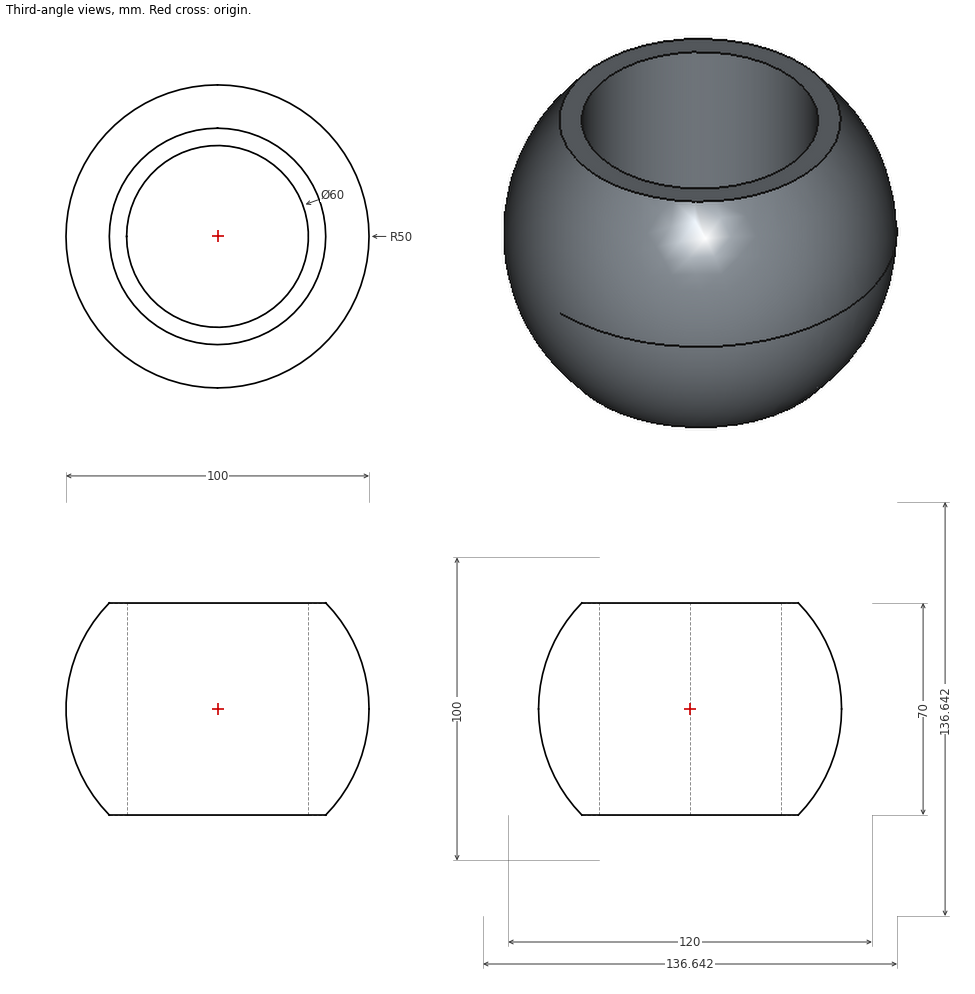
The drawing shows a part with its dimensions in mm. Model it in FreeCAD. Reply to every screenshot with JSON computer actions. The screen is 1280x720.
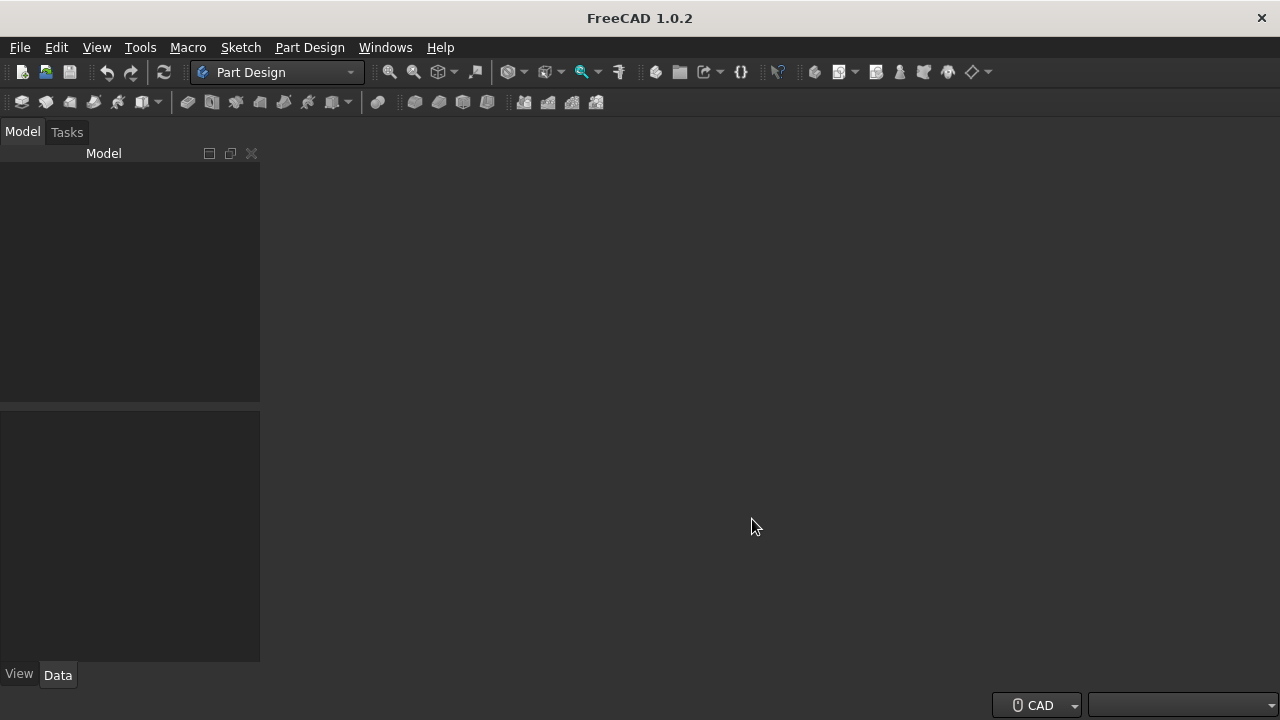
{"action": "left_click", "coordinate": [22, 72]}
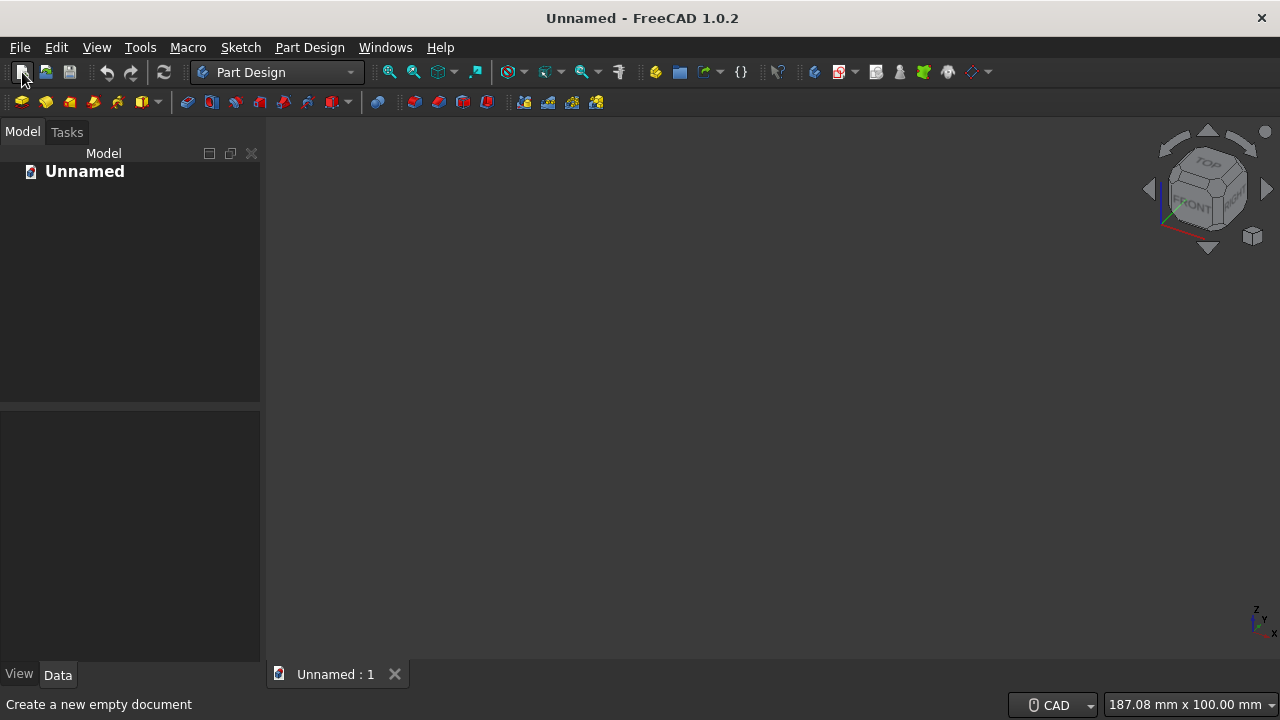
{"action": "left_click", "coordinate": [840, 72]}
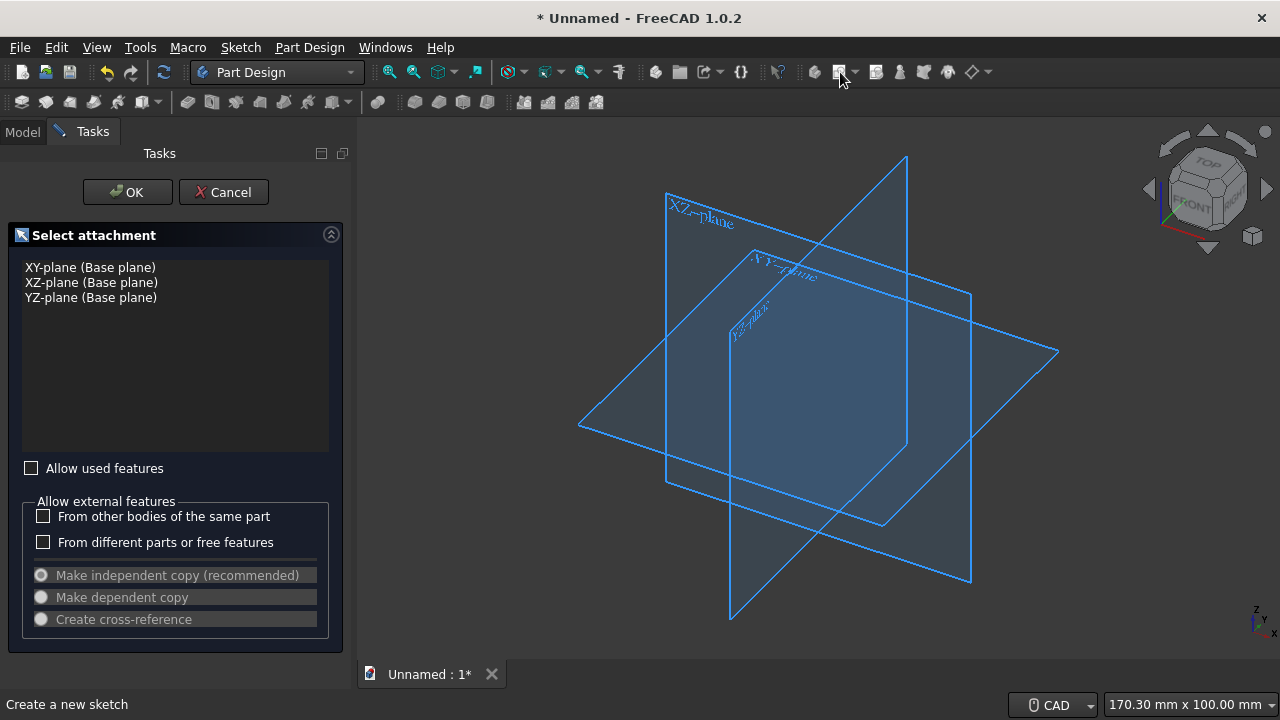
{"action": "left_click", "coordinate": [82, 268]}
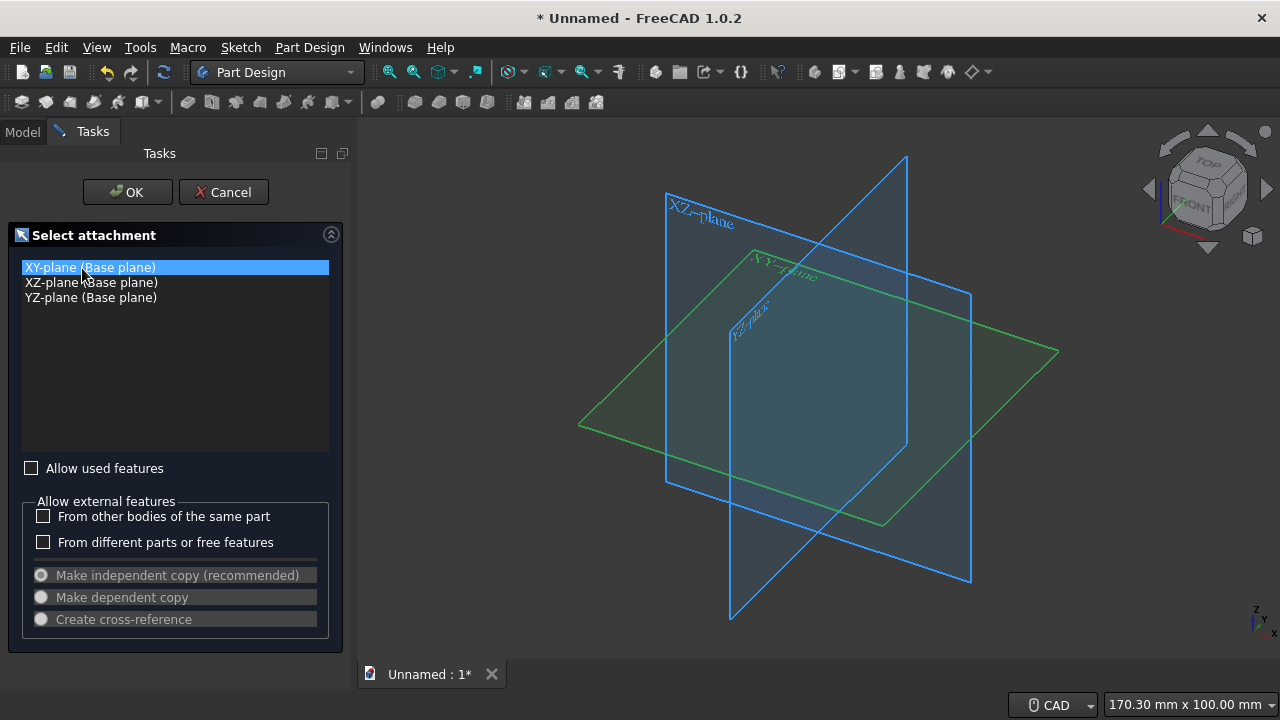
{"action": "left_click", "coordinate": [128, 192]}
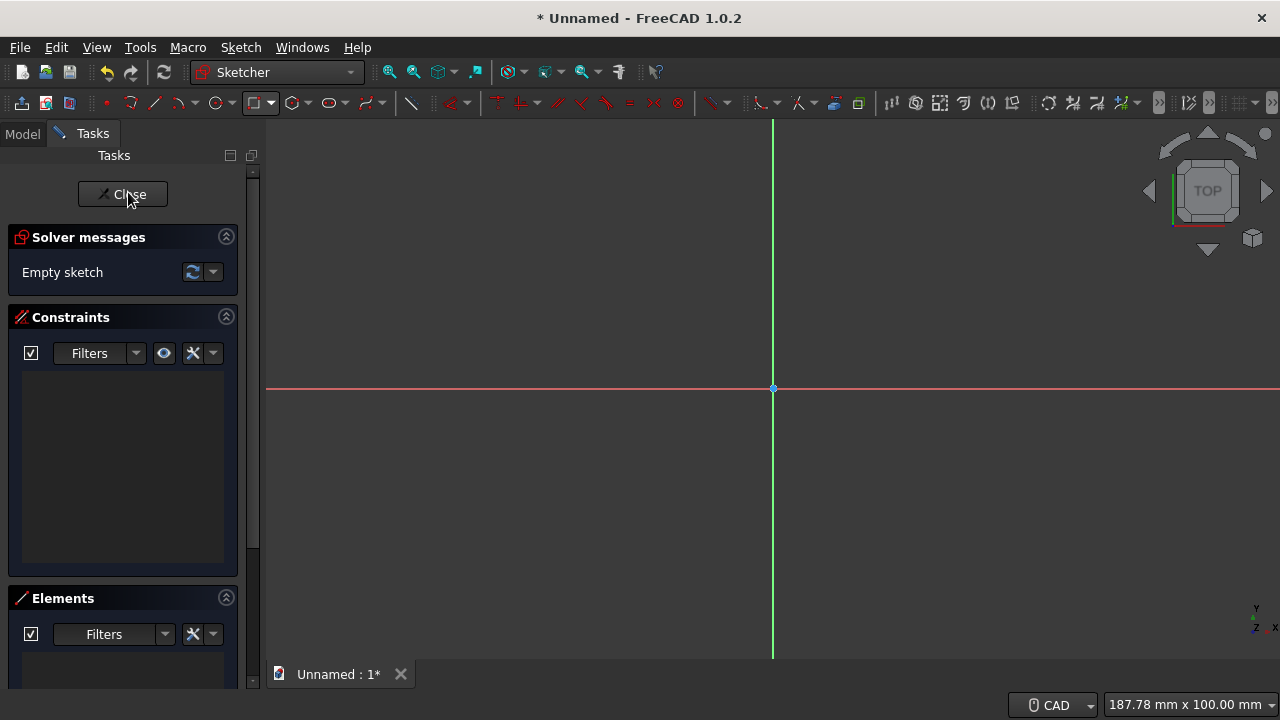
{"action": "scroll", "coordinate": [294, 389], "scroll_direction": "down", "scroll_amount": 2}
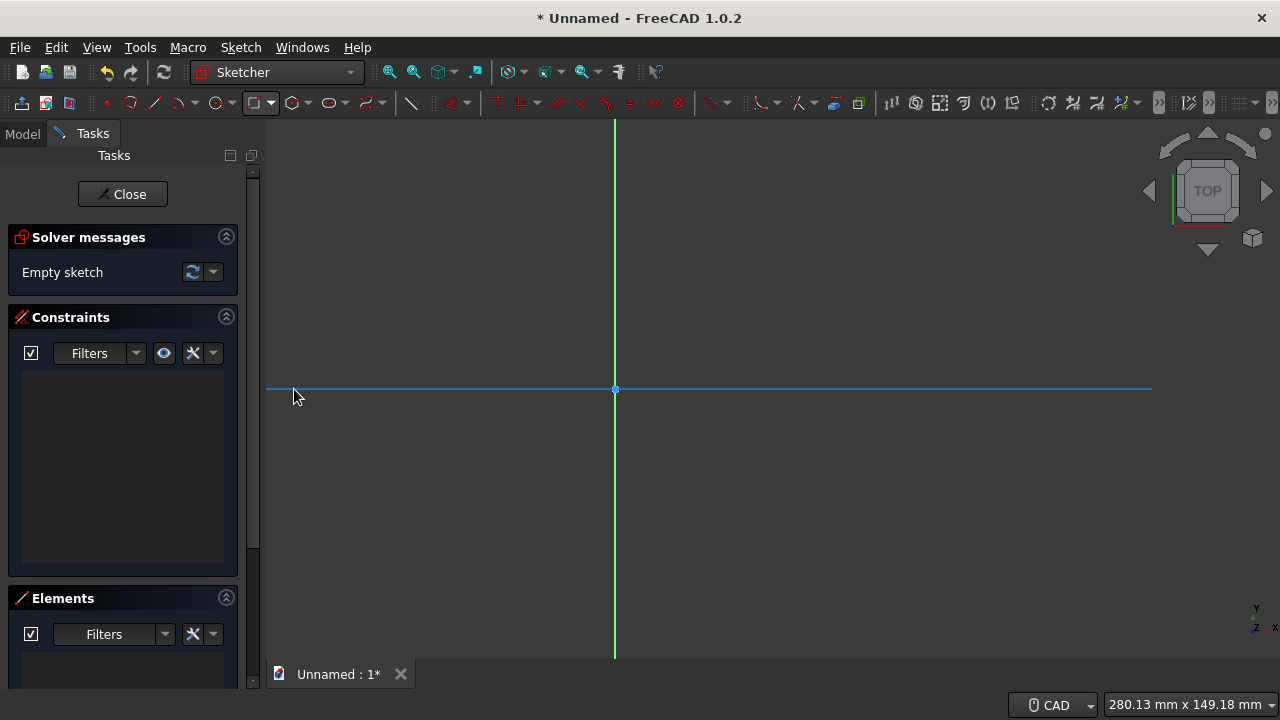
{"action": "left_click", "coordinate": [156, 104]}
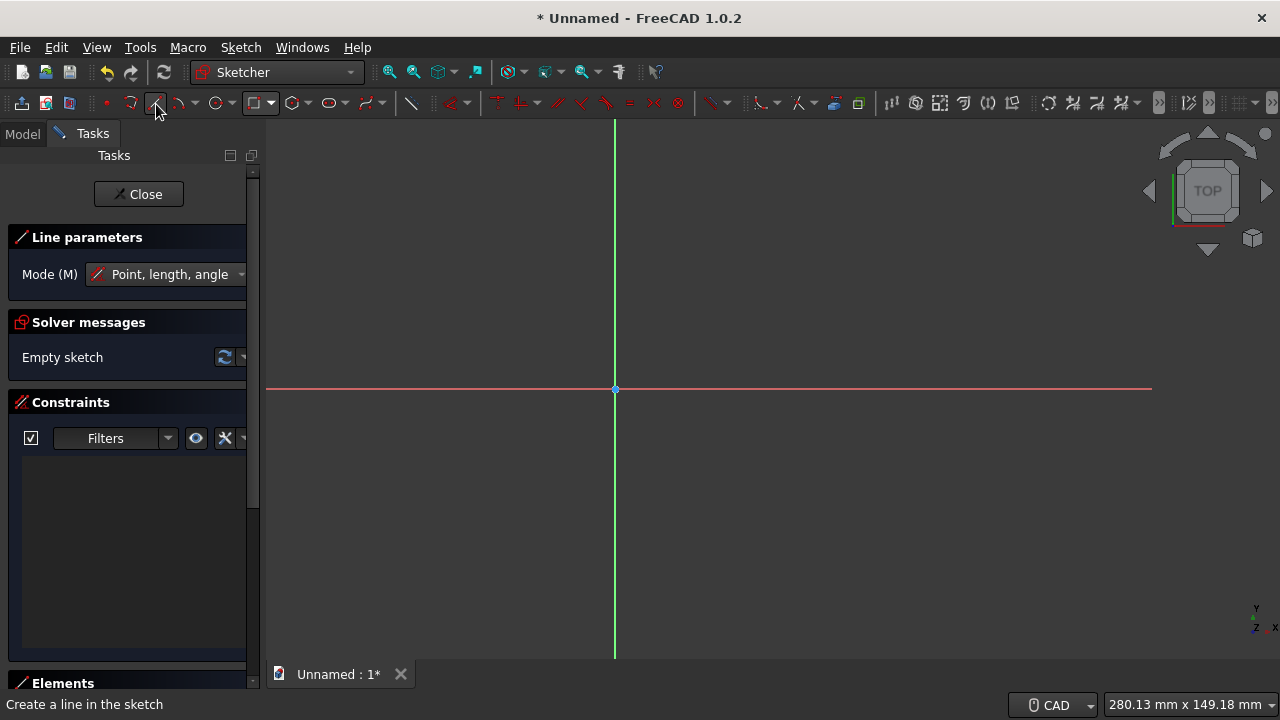
{"action": "left_click", "coordinate": [615, 208]}
{"action": "left_click", "coordinate": [624, 570]}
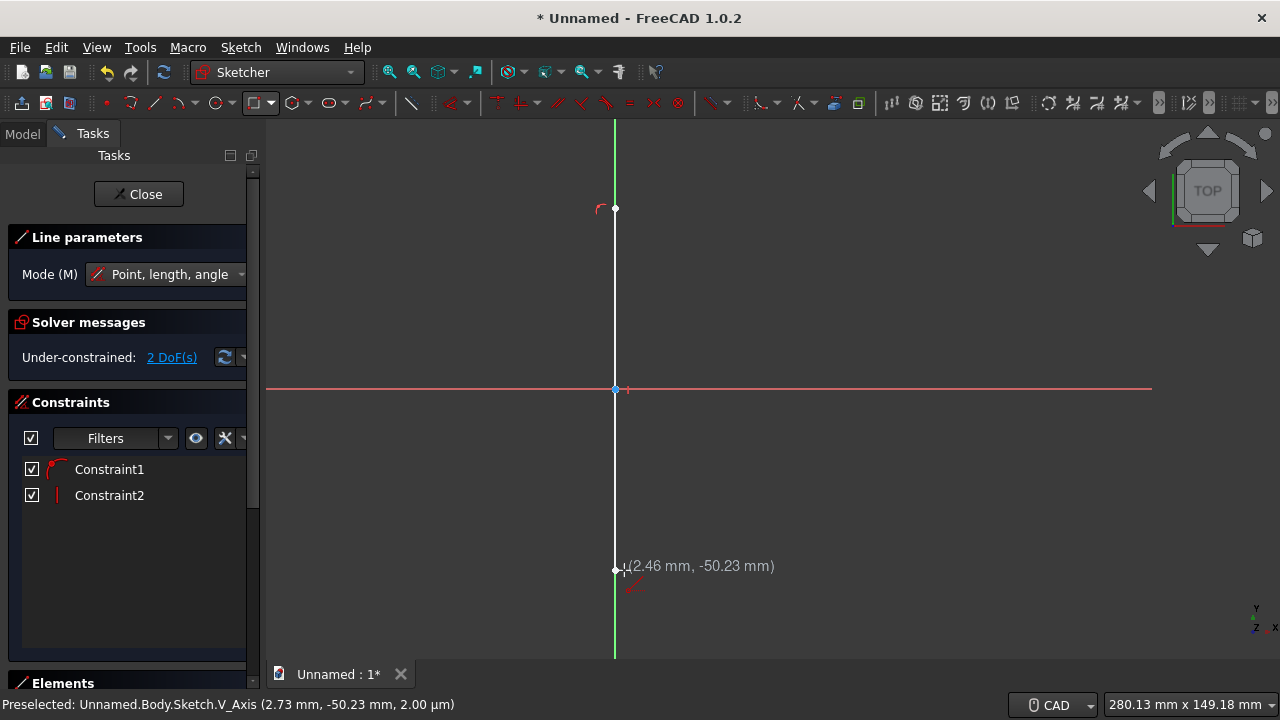
{"action": "left_click", "coordinate": [198, 104]}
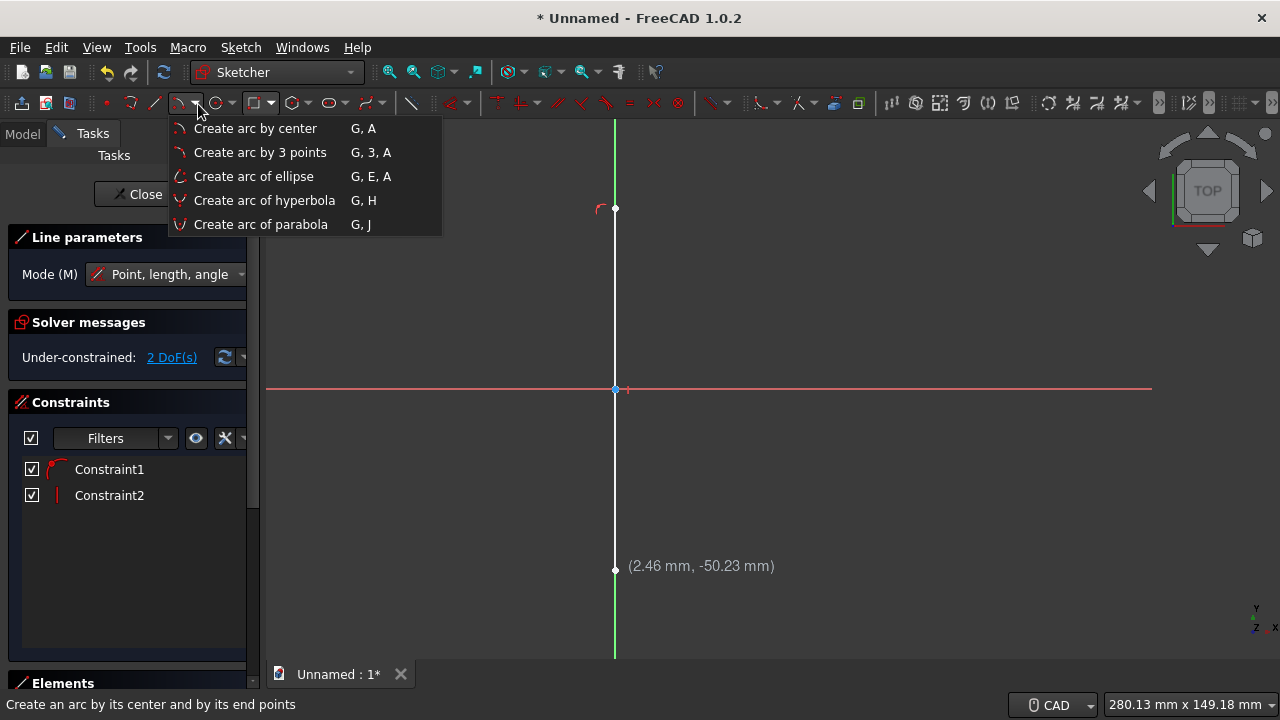
{"action": "left_click", "coordinate": [306, 152]}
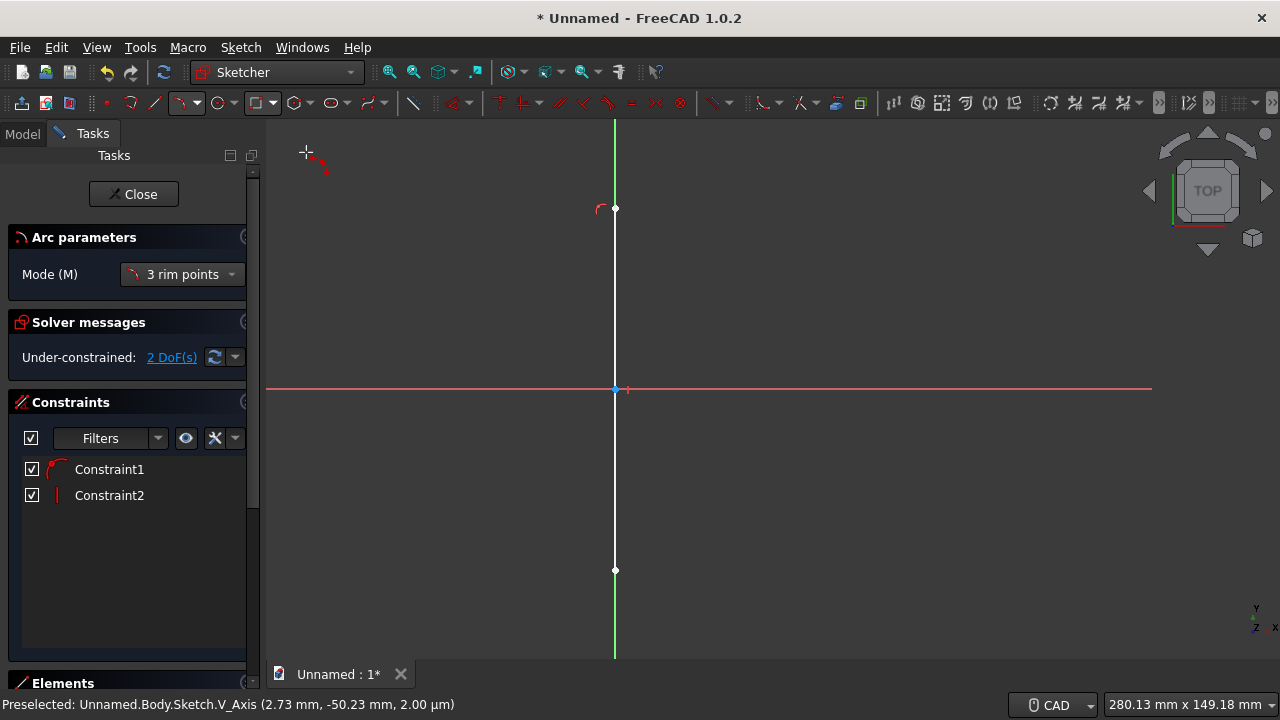
{"action": "left_click", "coordinate": [615, 571]}
{"action": "left_click", "coordinate": [615, 209]}
{"action": "left_click", "coordinate": [787, 445]}
{"action": "key", "text": "Escape"}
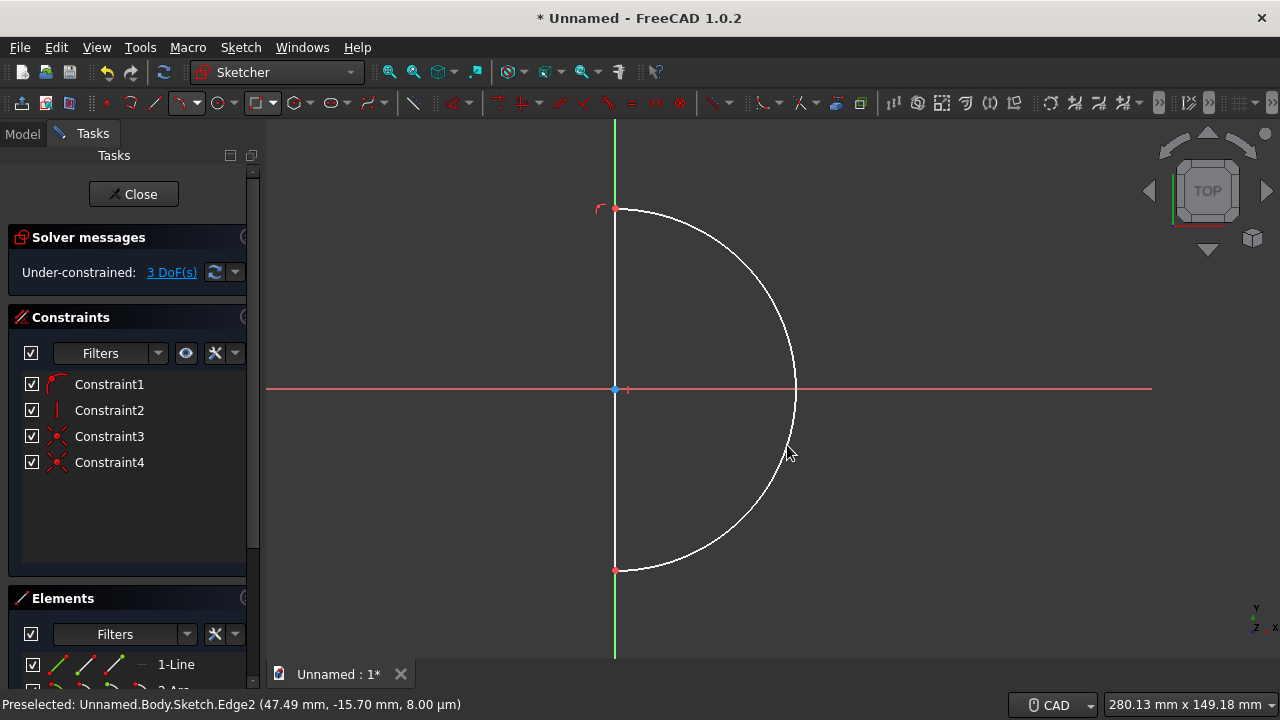
{"action": "left_click_drag", "start_coordinate": [605, 379], "coordinate": [625, 400]}